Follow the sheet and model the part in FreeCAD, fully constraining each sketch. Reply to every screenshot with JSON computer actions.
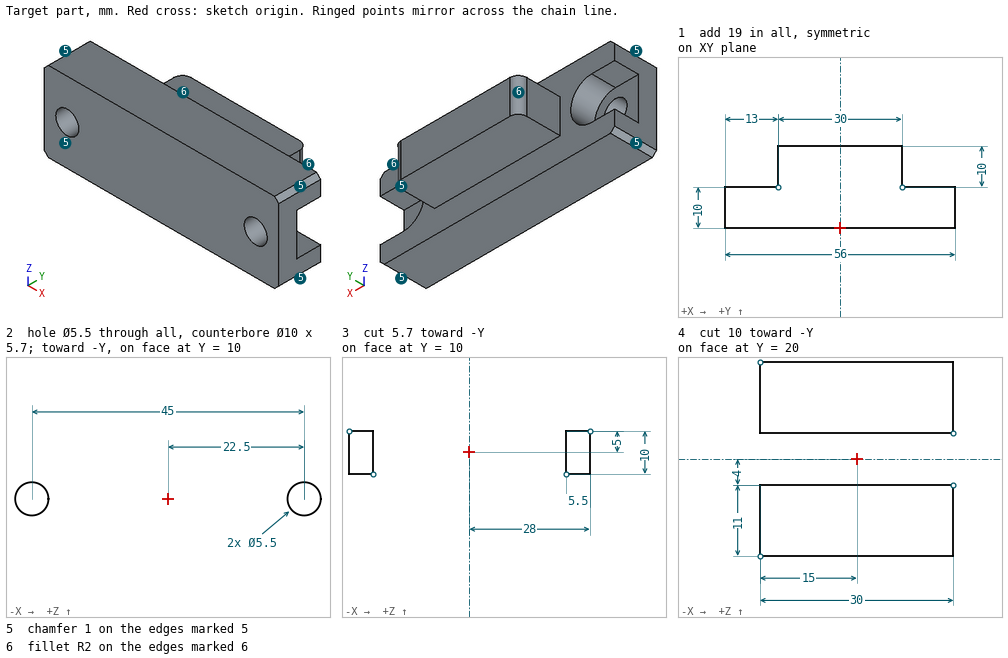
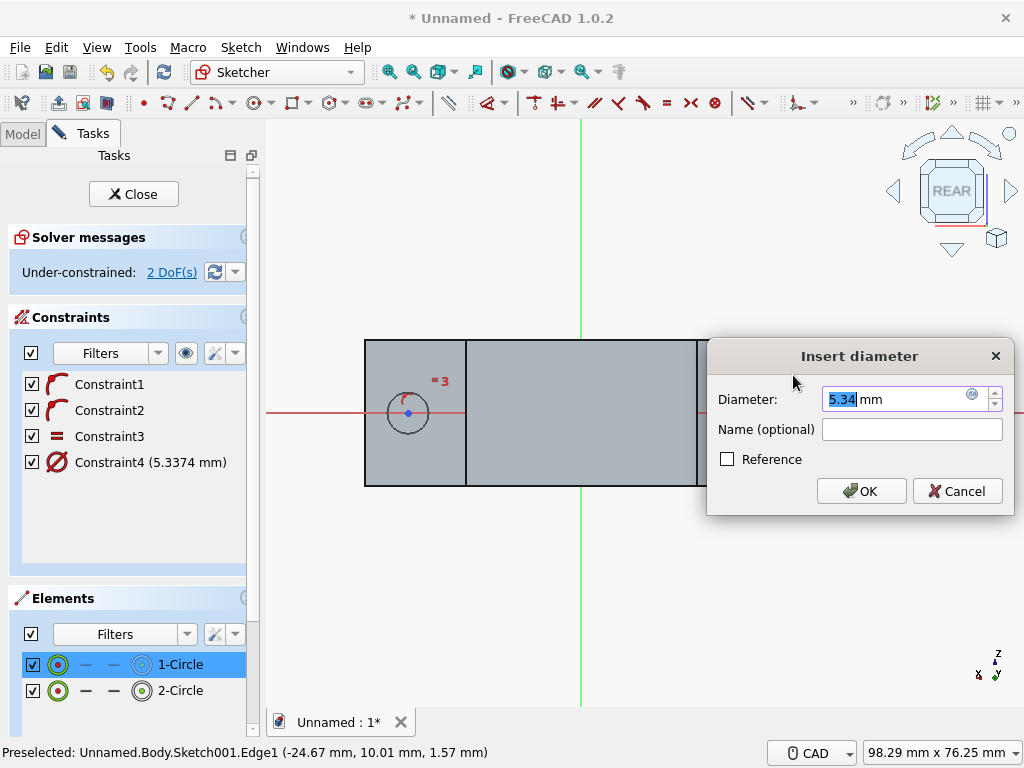
{"action": "type", "text": "5.5"}
{"action": "key", "text": "Return"}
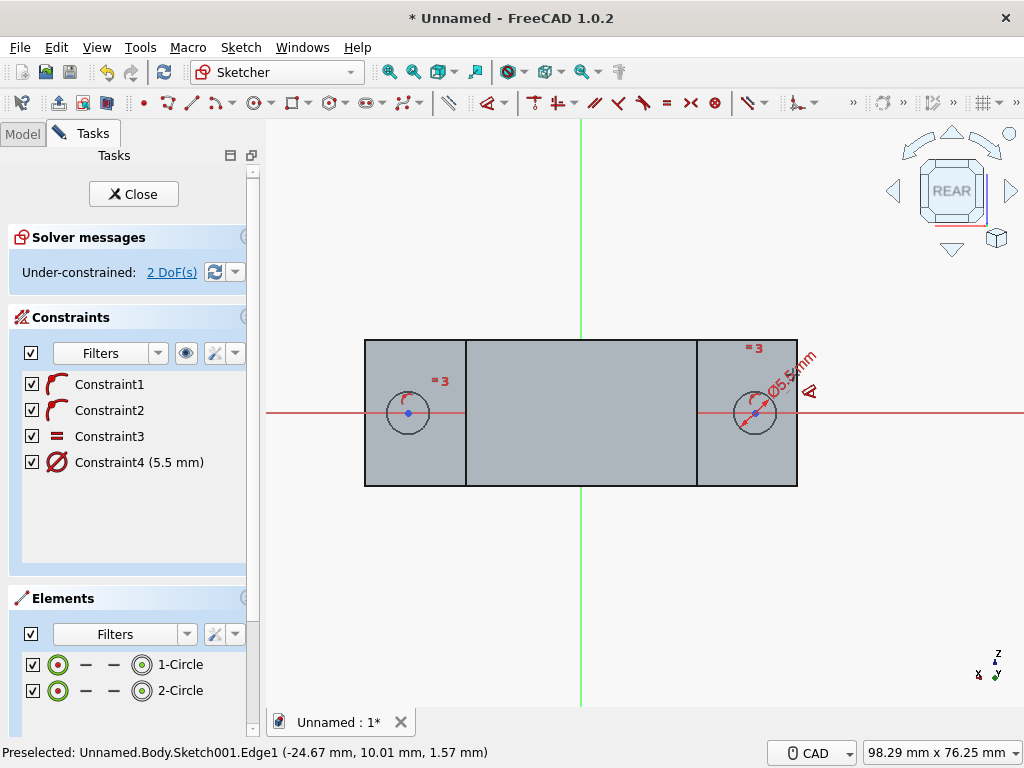
{"action": "left_click", "coordinate": [755, 413]}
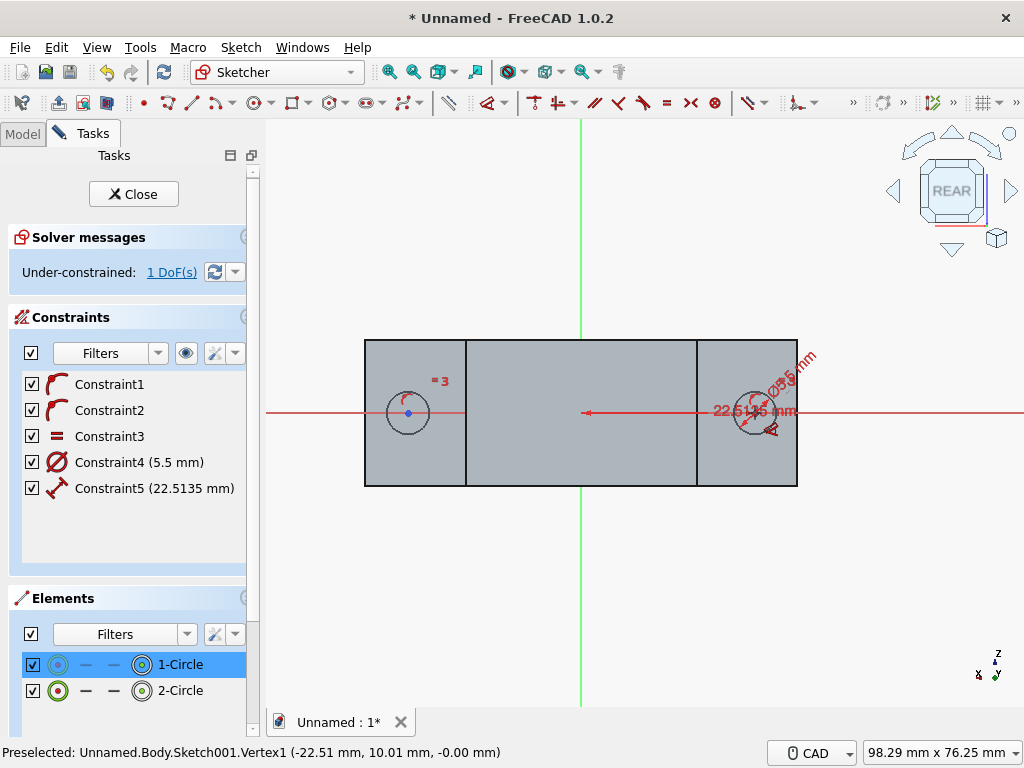
{"action": "left_click", "coordinate": [408, 413]}
{"action": "left_click", "coordinate": [502, 447]}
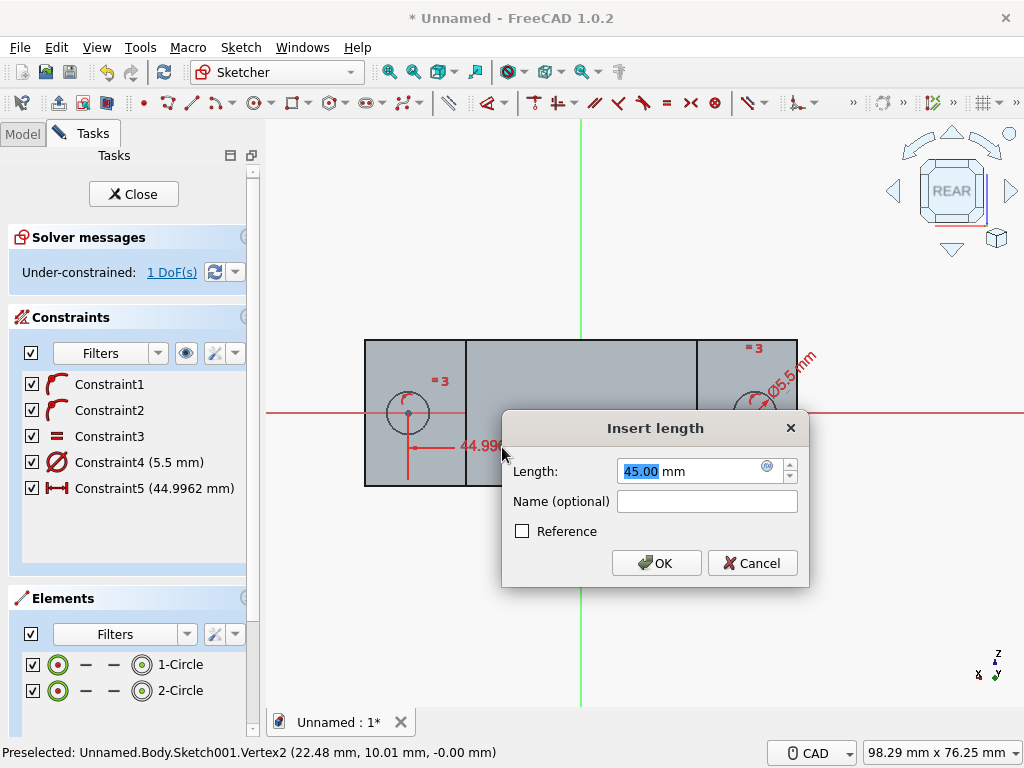
{"action": "type", "text": "45"}
{"action": "key", "text": "Return"}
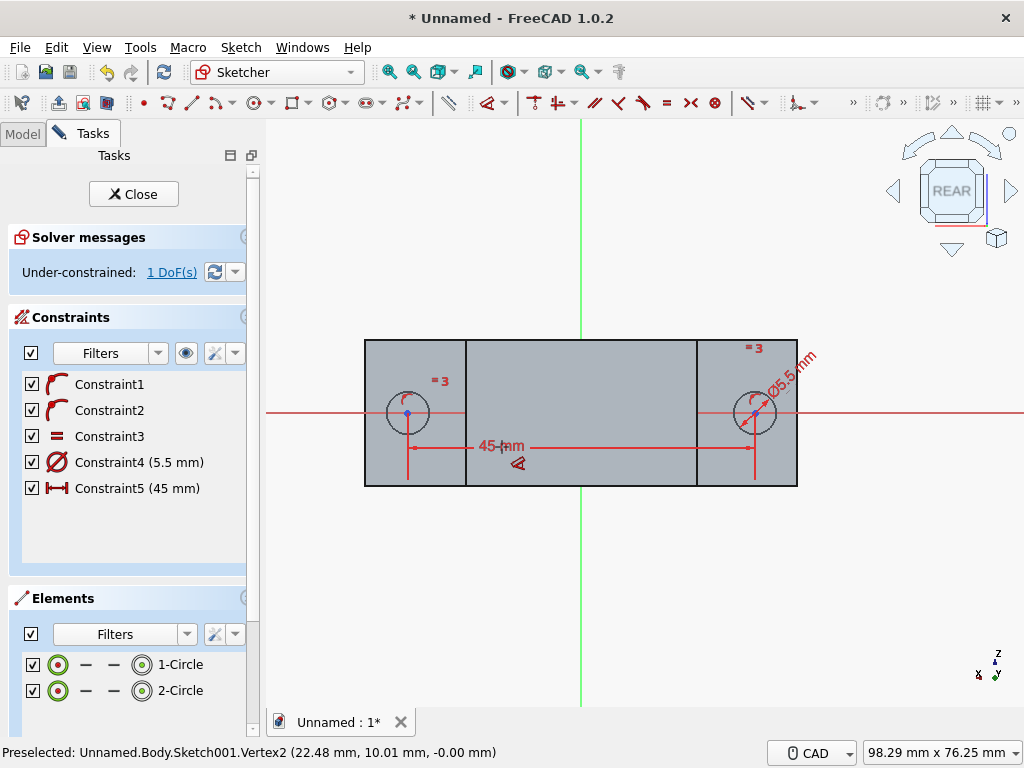
{"action": "left_click", "coordinate": [755, 413]}
{"action": "left_click", "coordinate": [668, 447]}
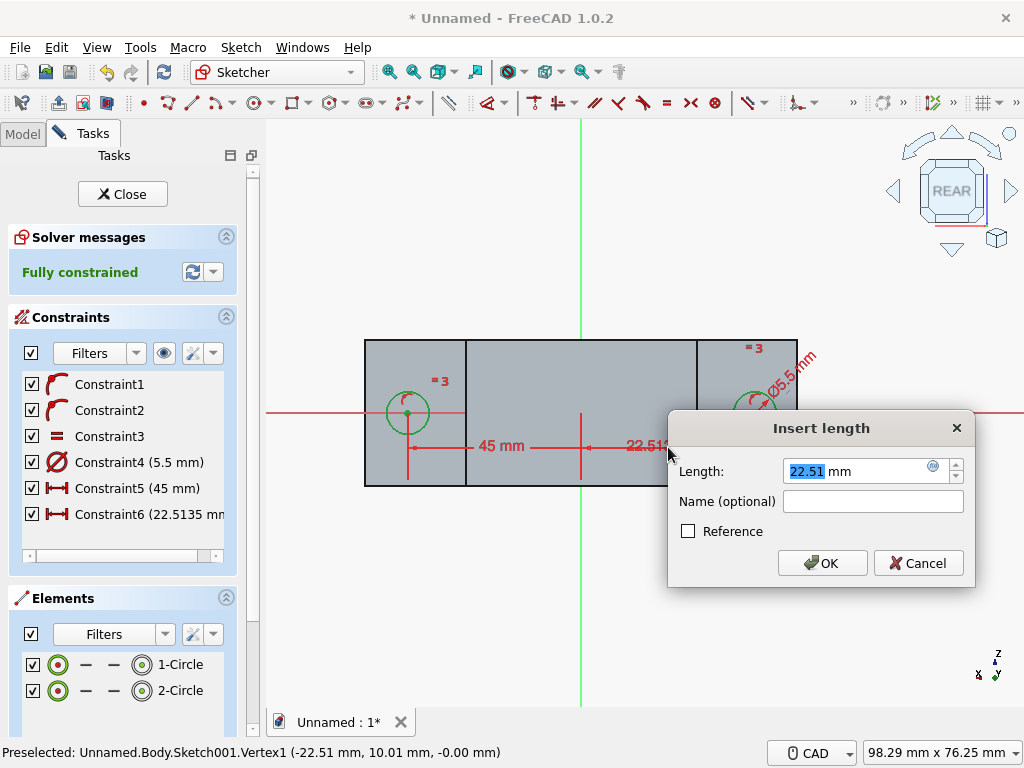
{"action": "type", "text": "22.5"}
{"action": "key", "text": "Return"}
{"action": "key", "text": "Escape"}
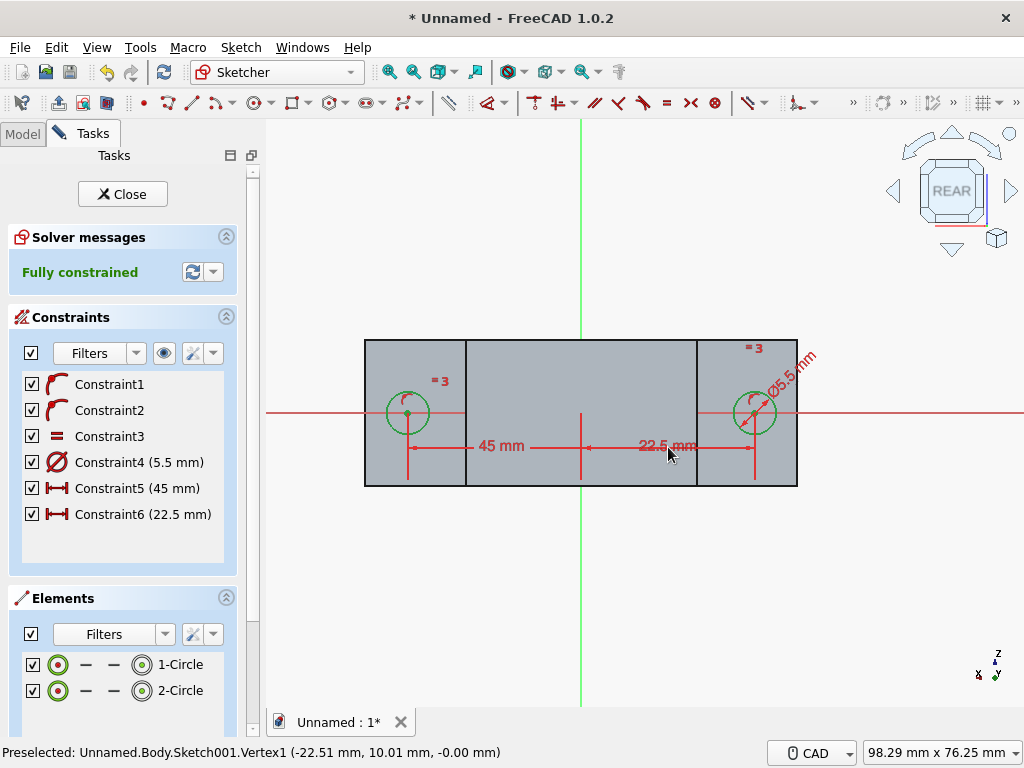
{"action": "left_click", "coordinate": [123, 194]}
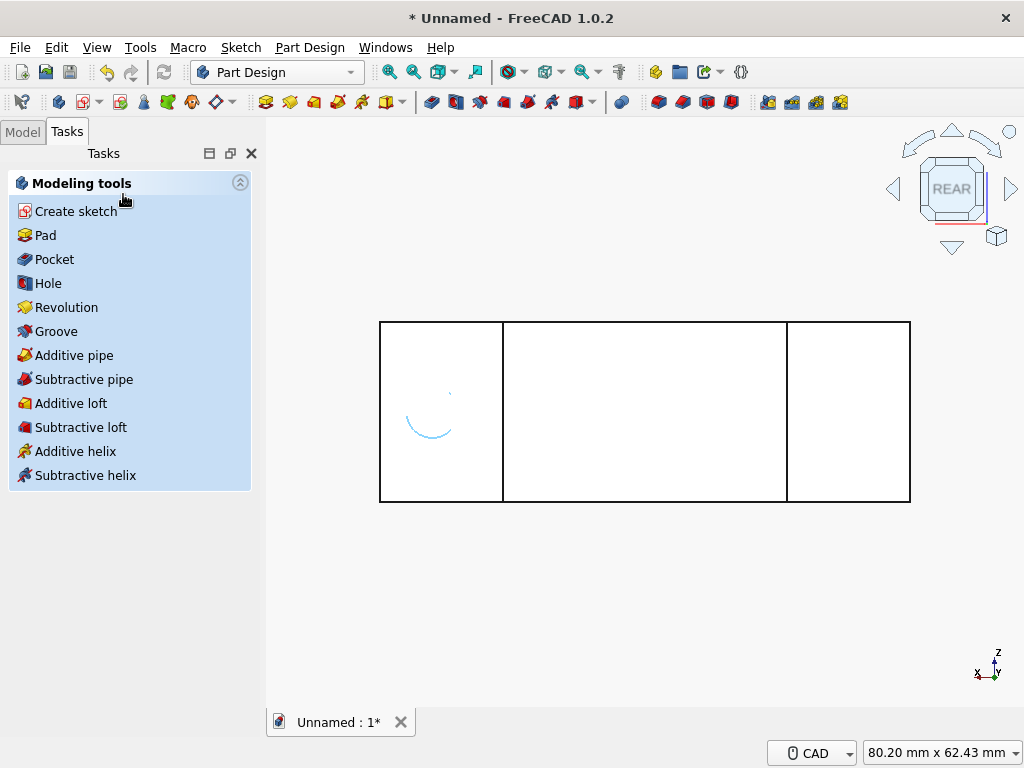
{"action": "left_click", "coordinate": [456, 102]}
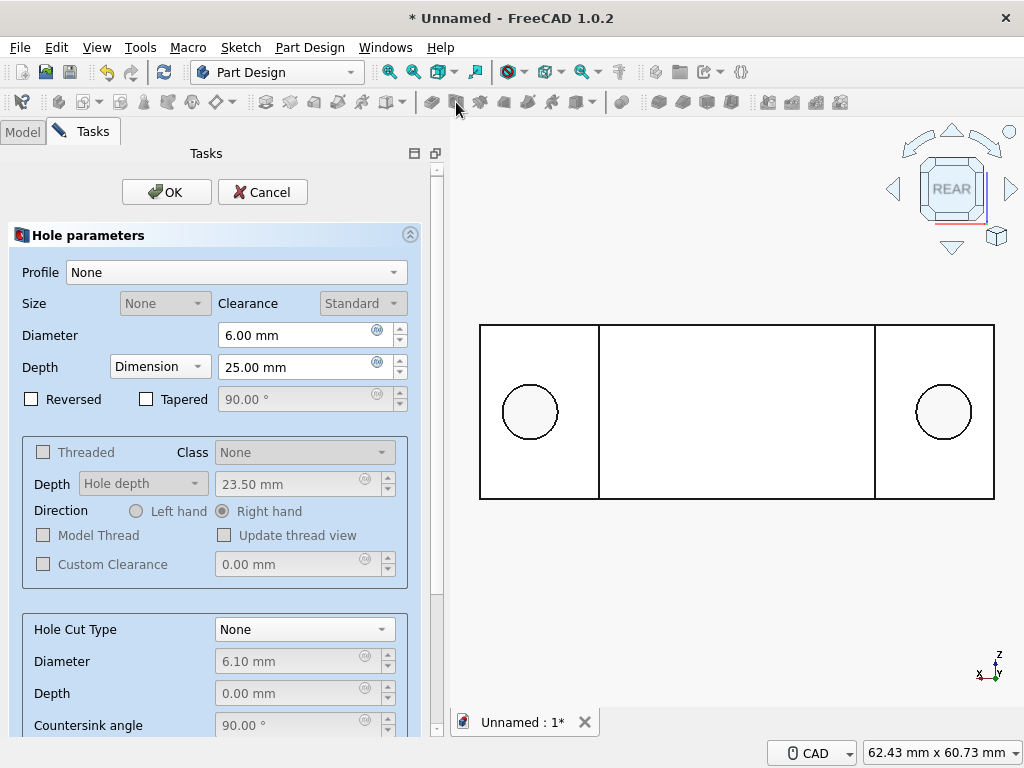
{"action": "triple_click", "coordinate": [305, 335]}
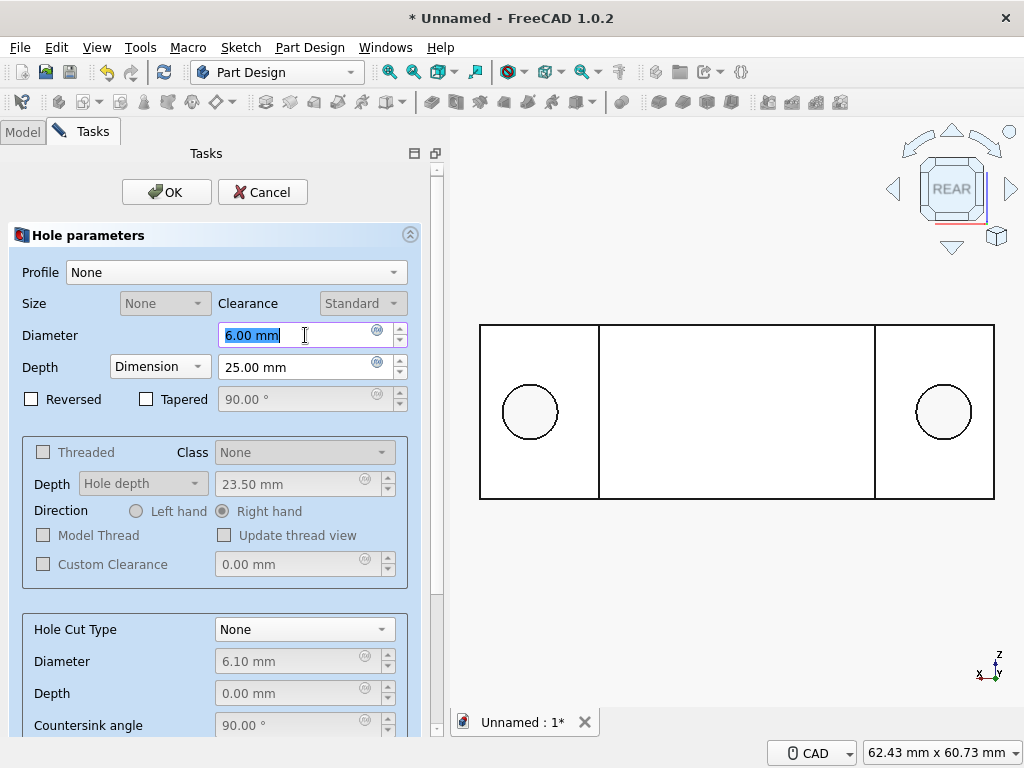
{"action": "type", "text": "5.5"}
{"action": "key", "text": "Tab"}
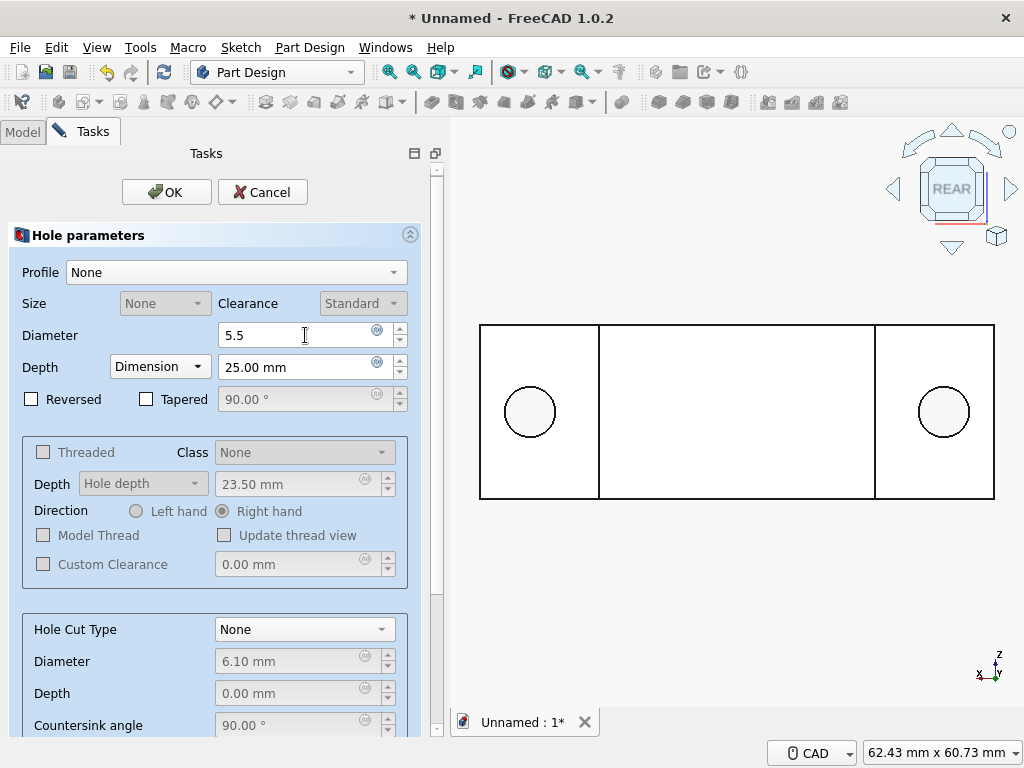
{"action": "left_click", "coordinate": [161, 366]}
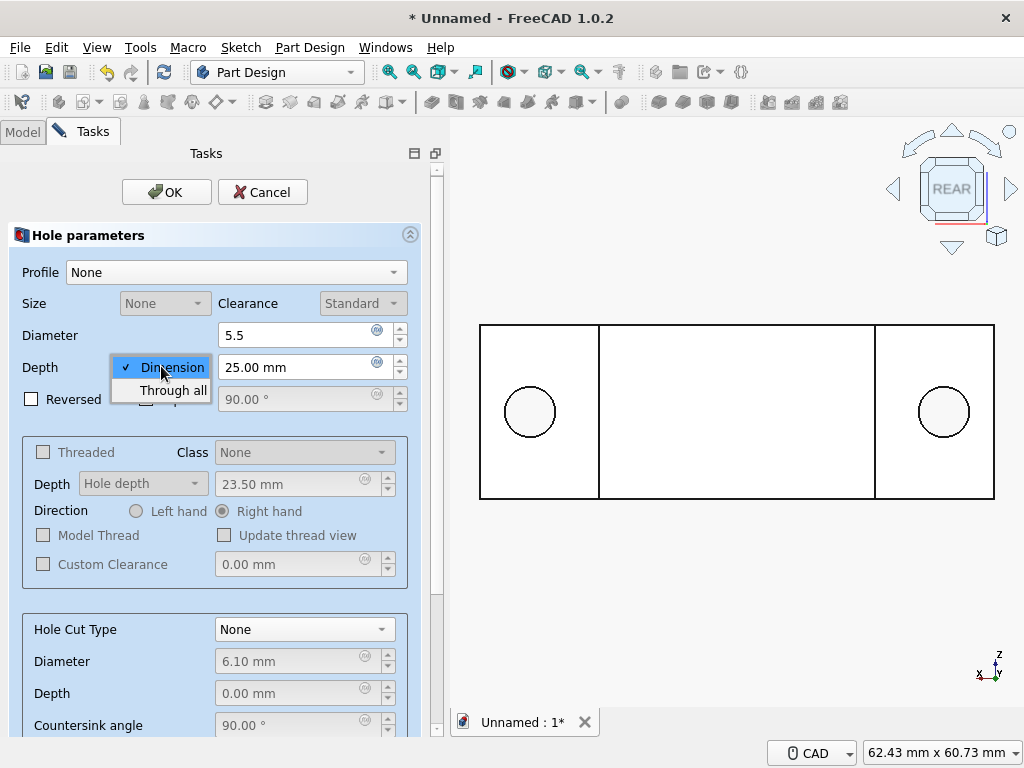
{"action": "left_click", "coordinate": [160, 390]}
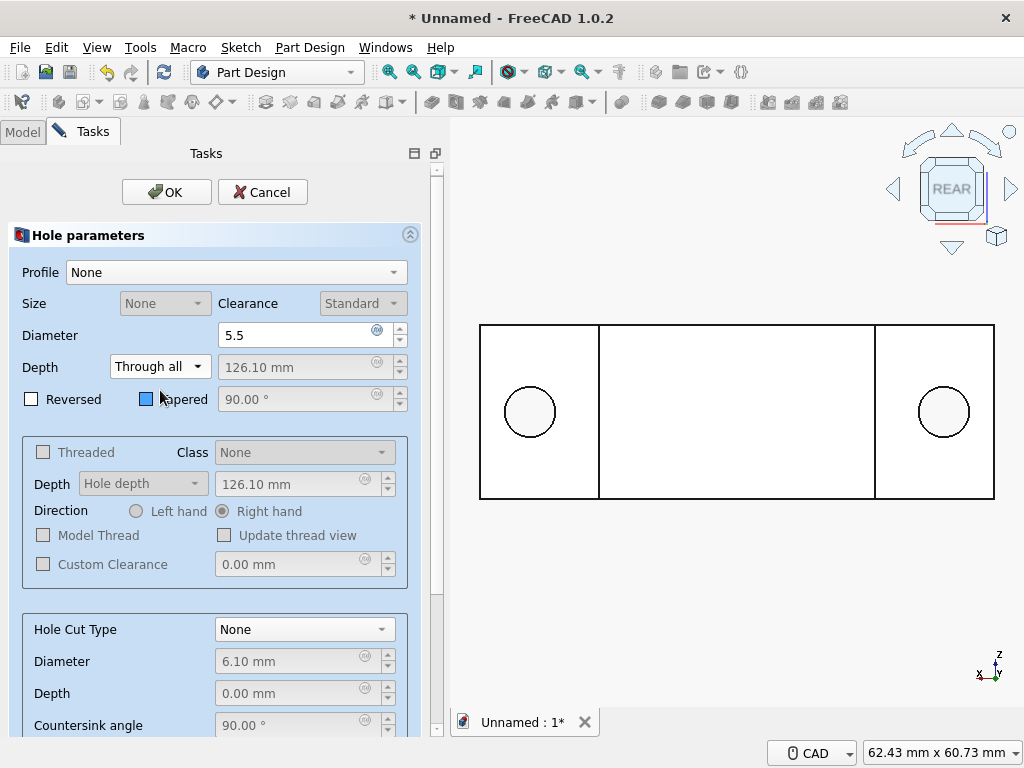
{"action": "left_click", "coordinate": [306, 630]}